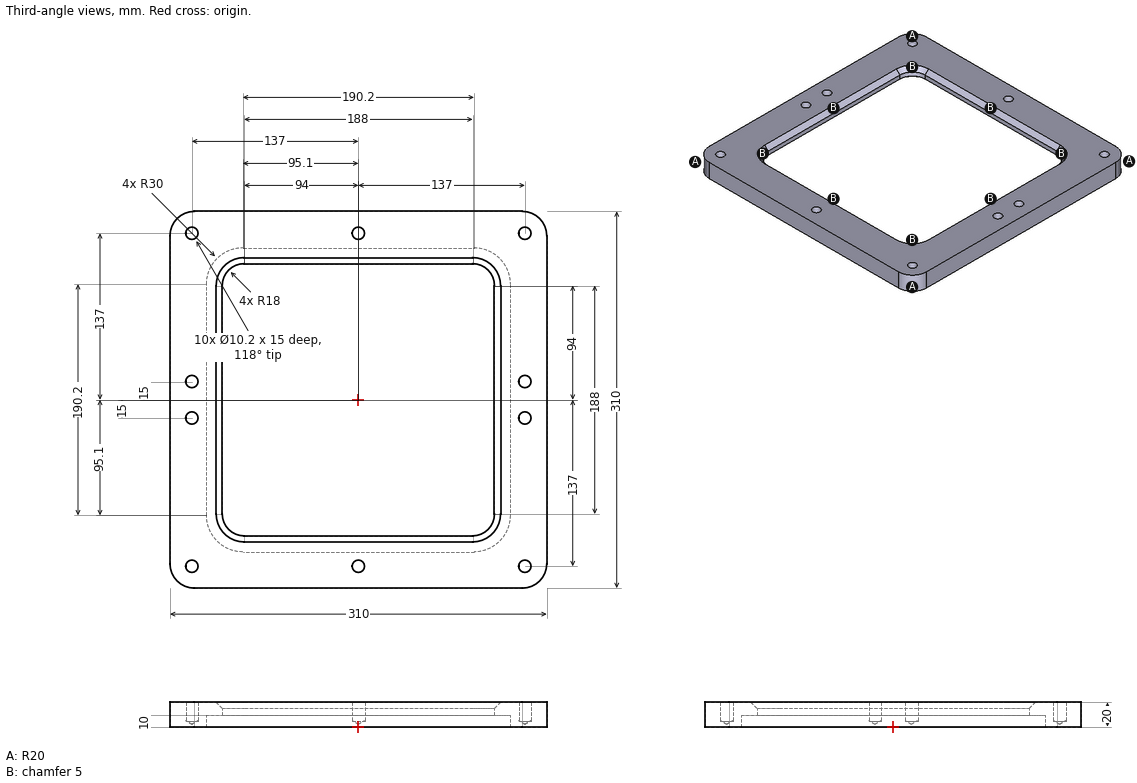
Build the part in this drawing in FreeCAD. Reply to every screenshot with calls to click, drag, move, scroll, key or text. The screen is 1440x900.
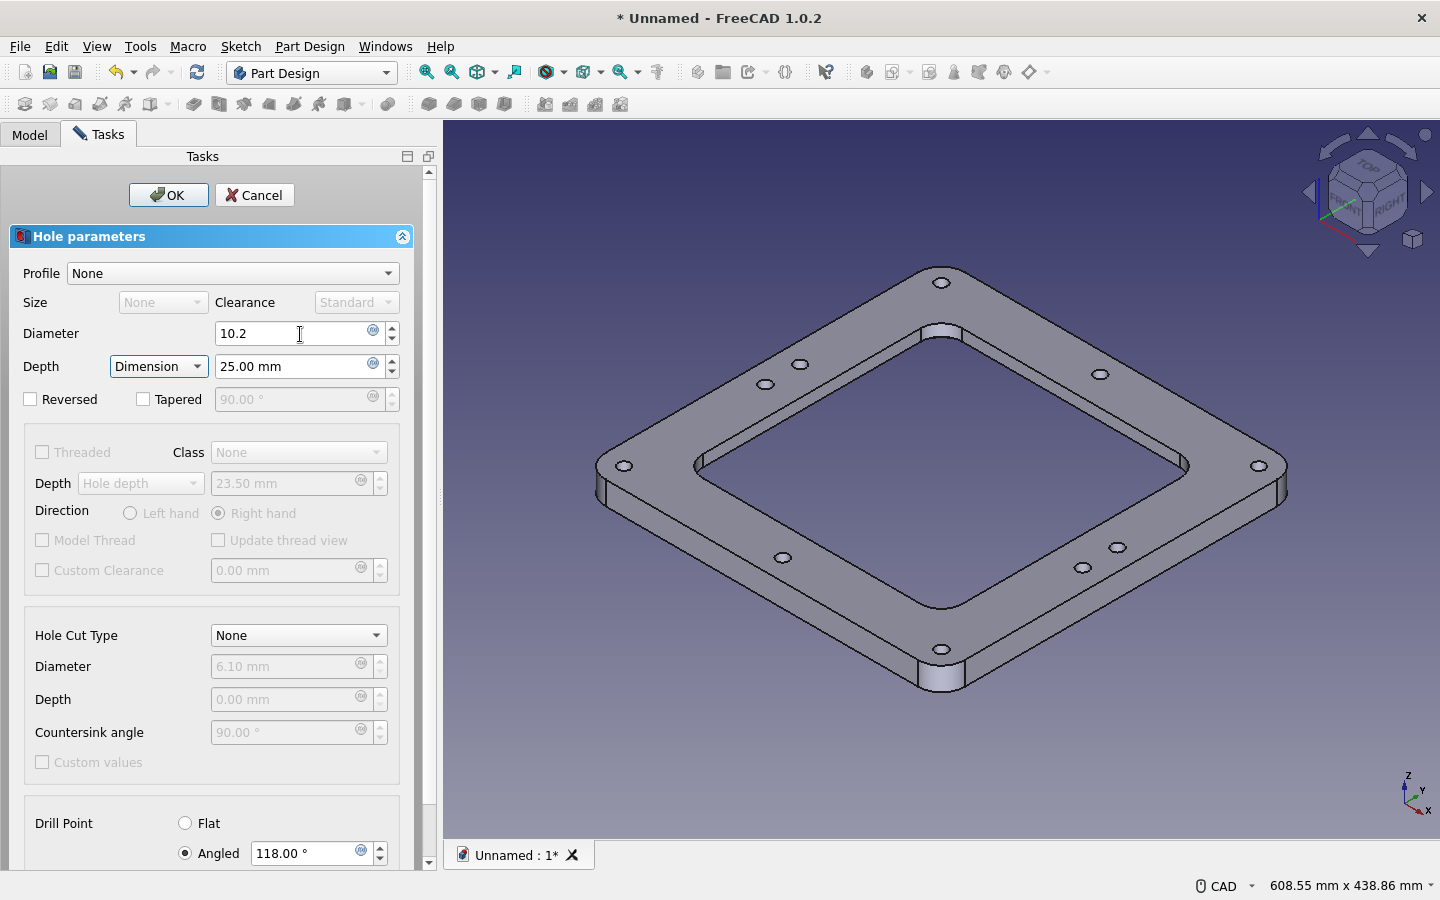
triple_click(300, 366)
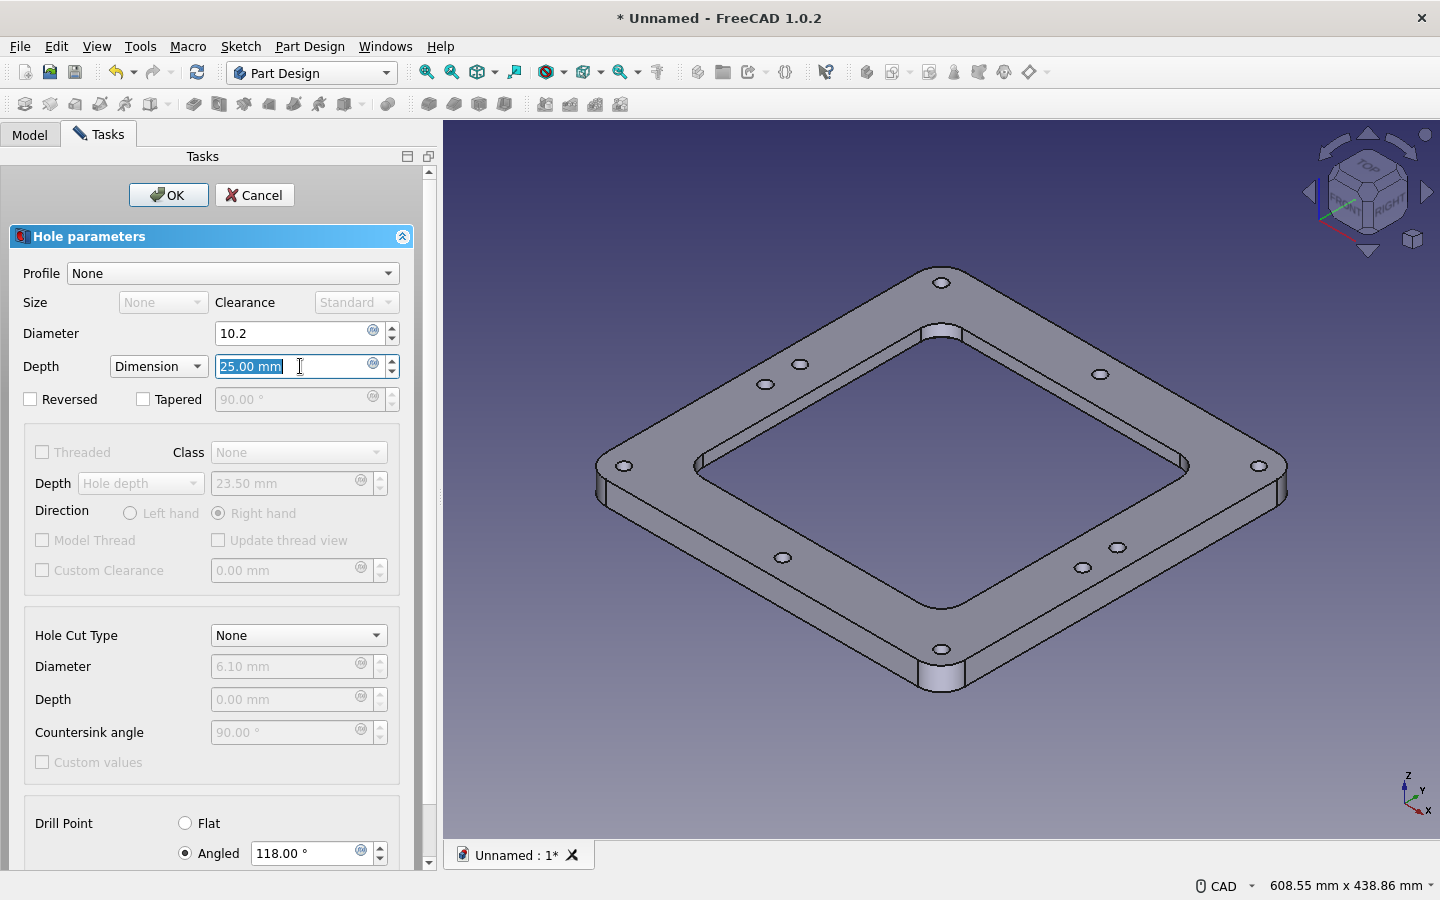
text(15)
key(Tab)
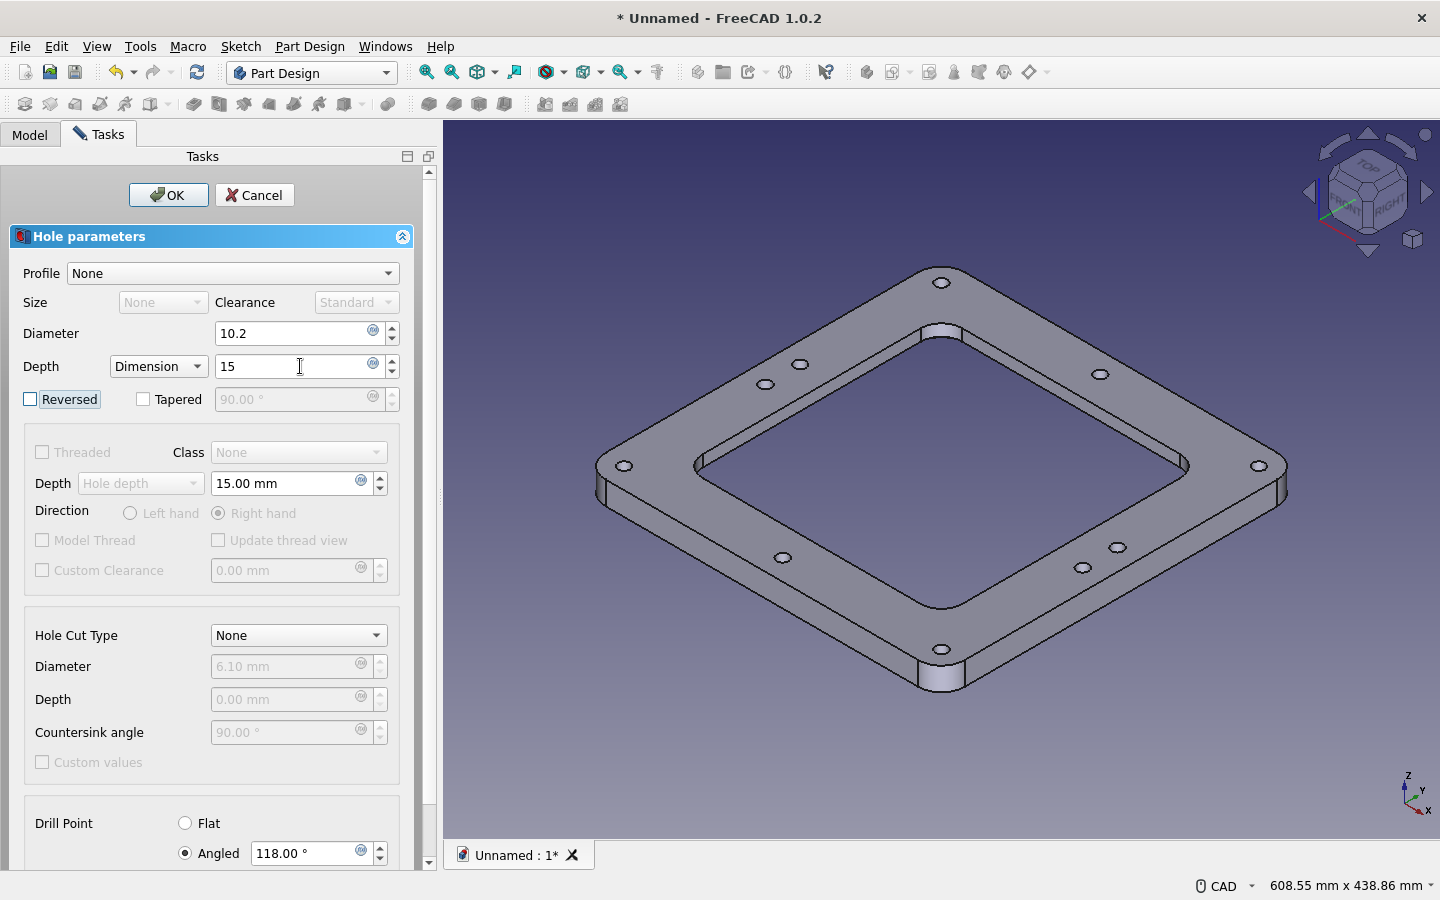
click(169, 195)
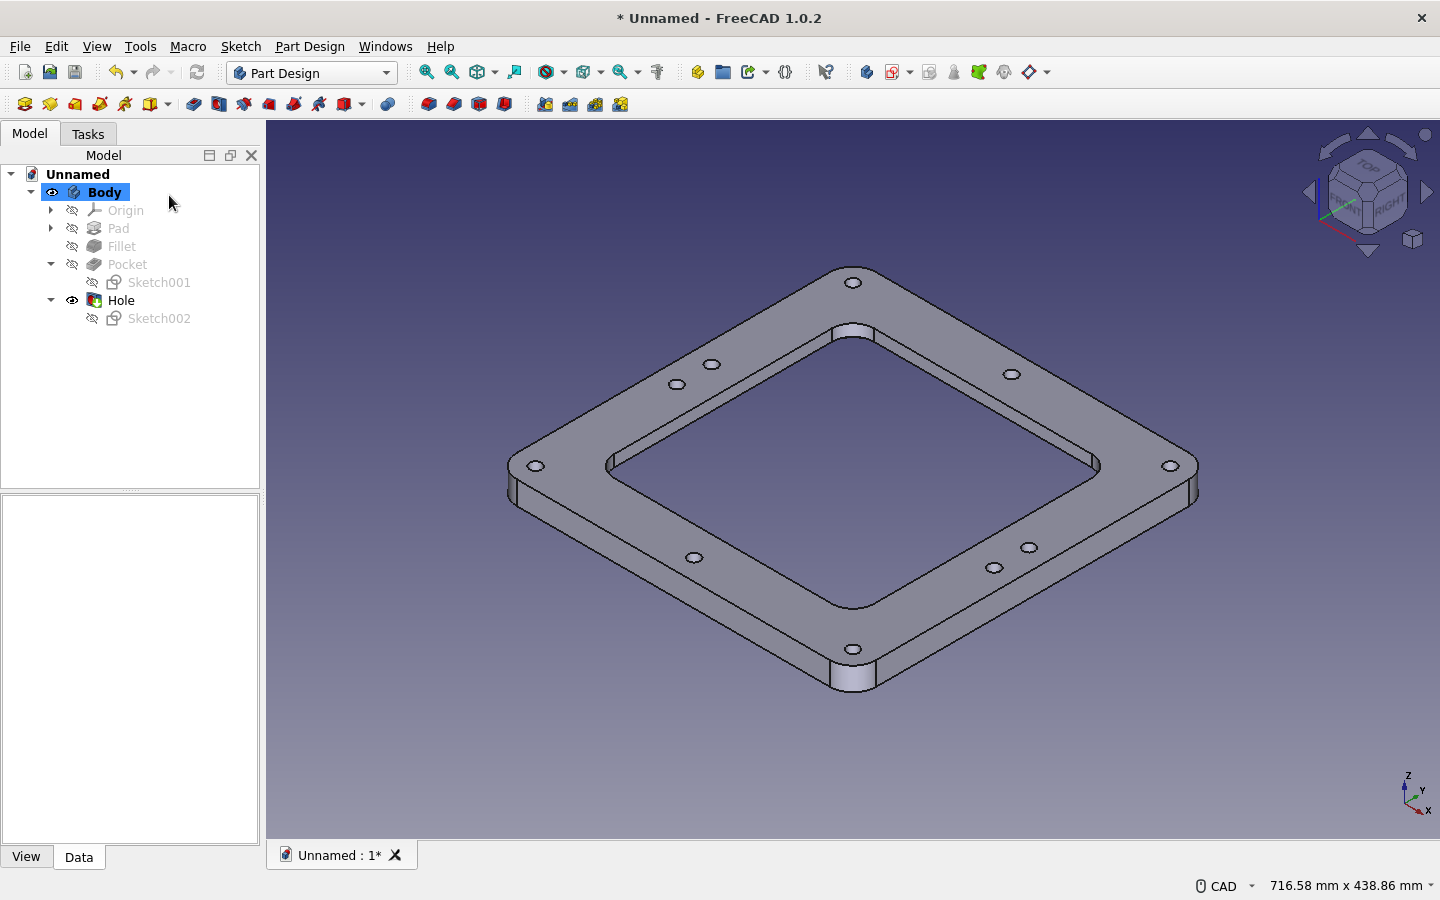
click(1100, 465)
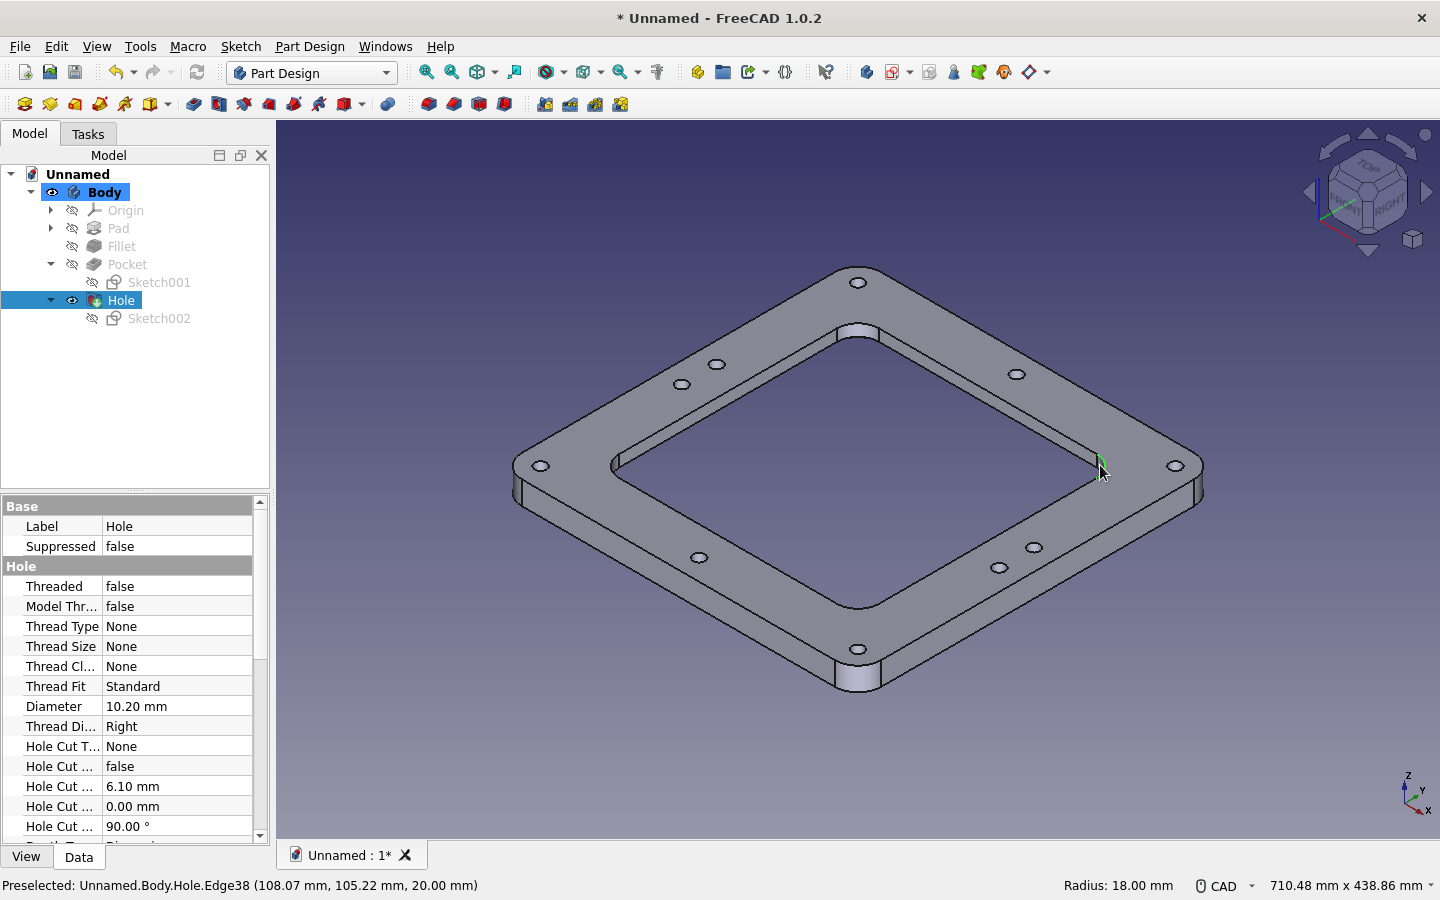
click(988, 390, ctrl)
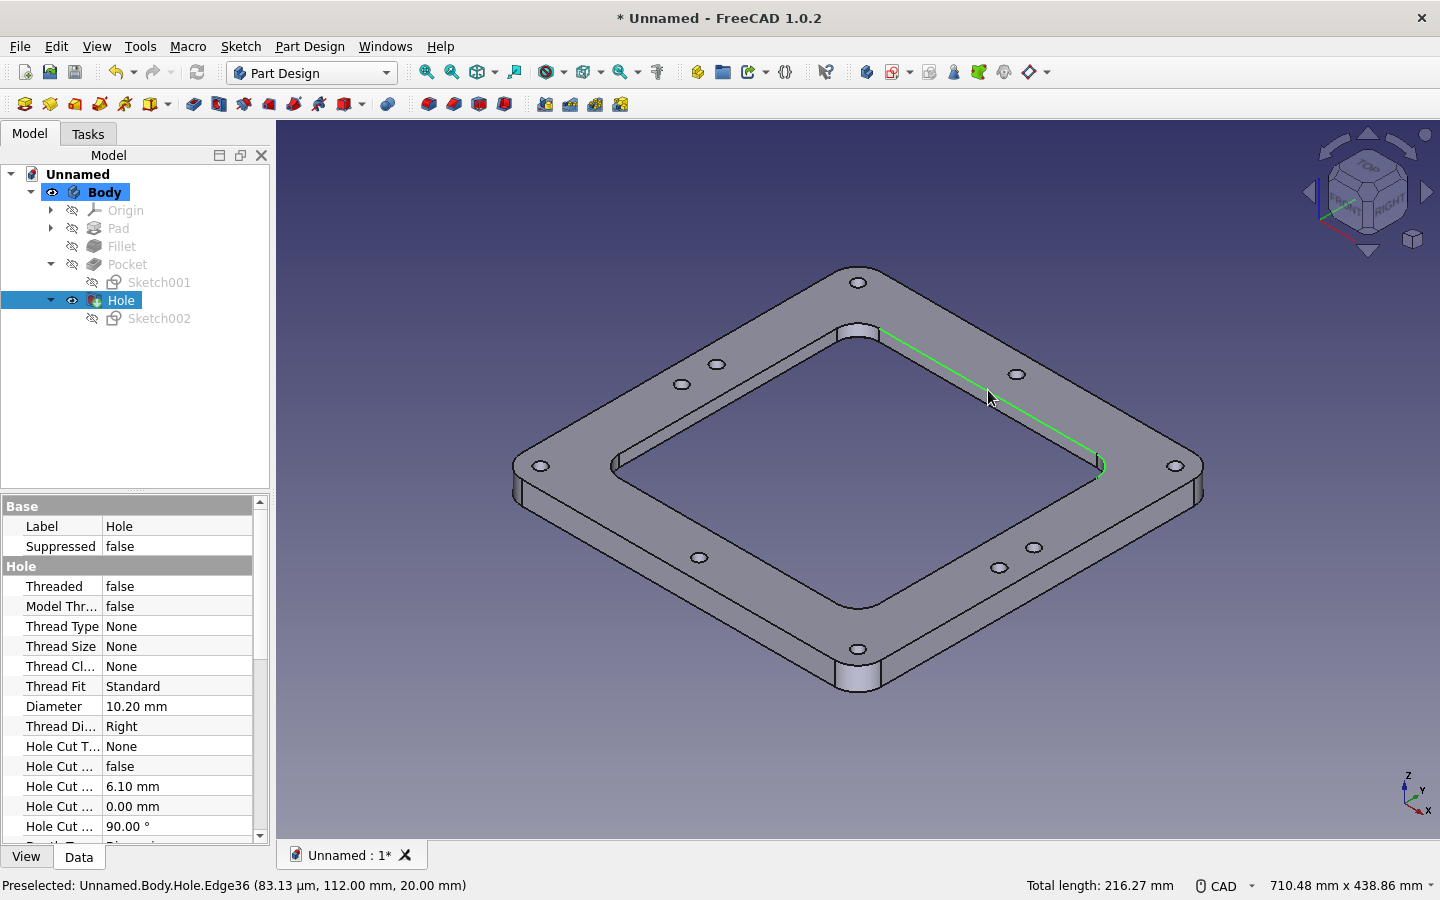
click(858, 322, ctrl)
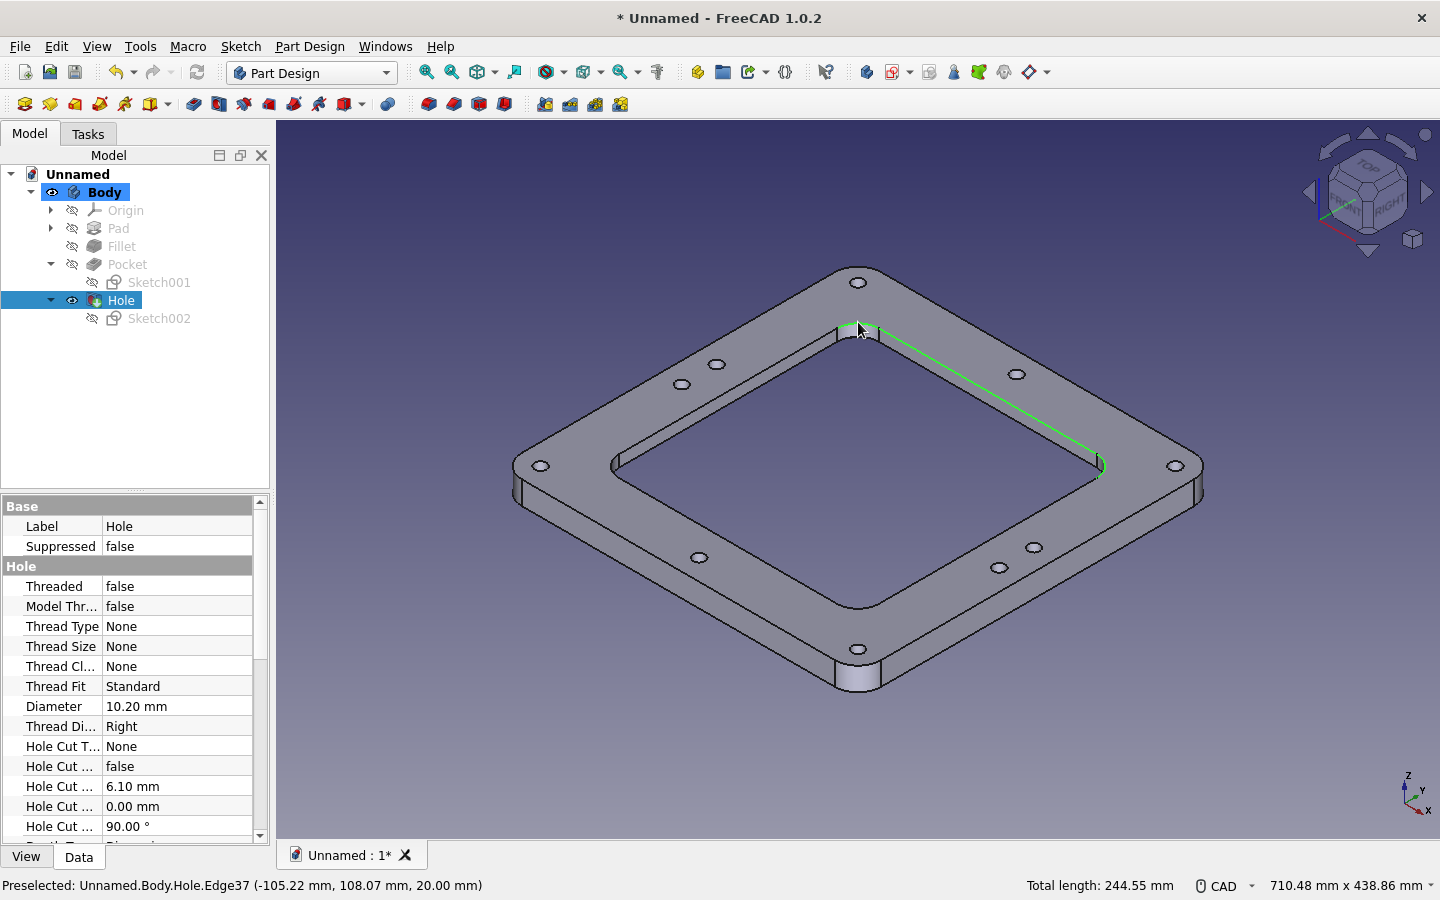
click(728, 390, ctrl)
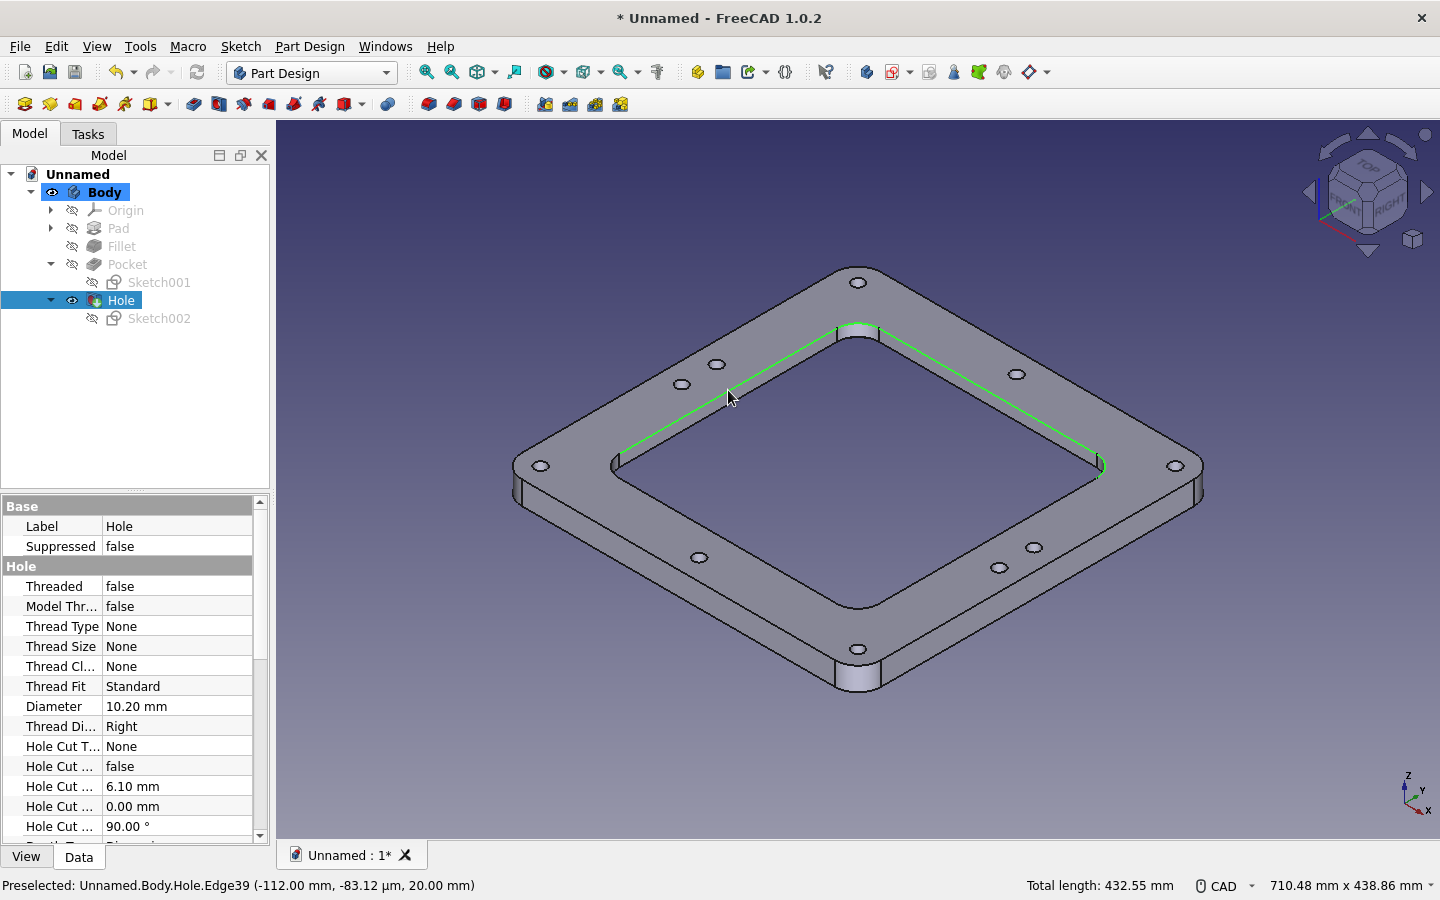
click(611, 465, ctrl)